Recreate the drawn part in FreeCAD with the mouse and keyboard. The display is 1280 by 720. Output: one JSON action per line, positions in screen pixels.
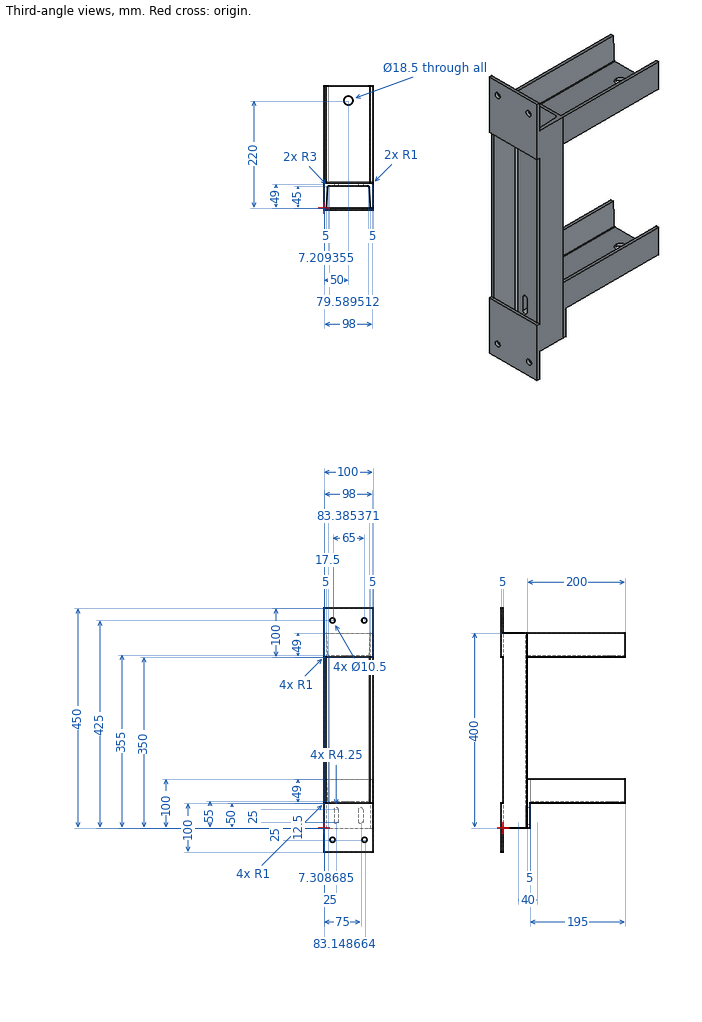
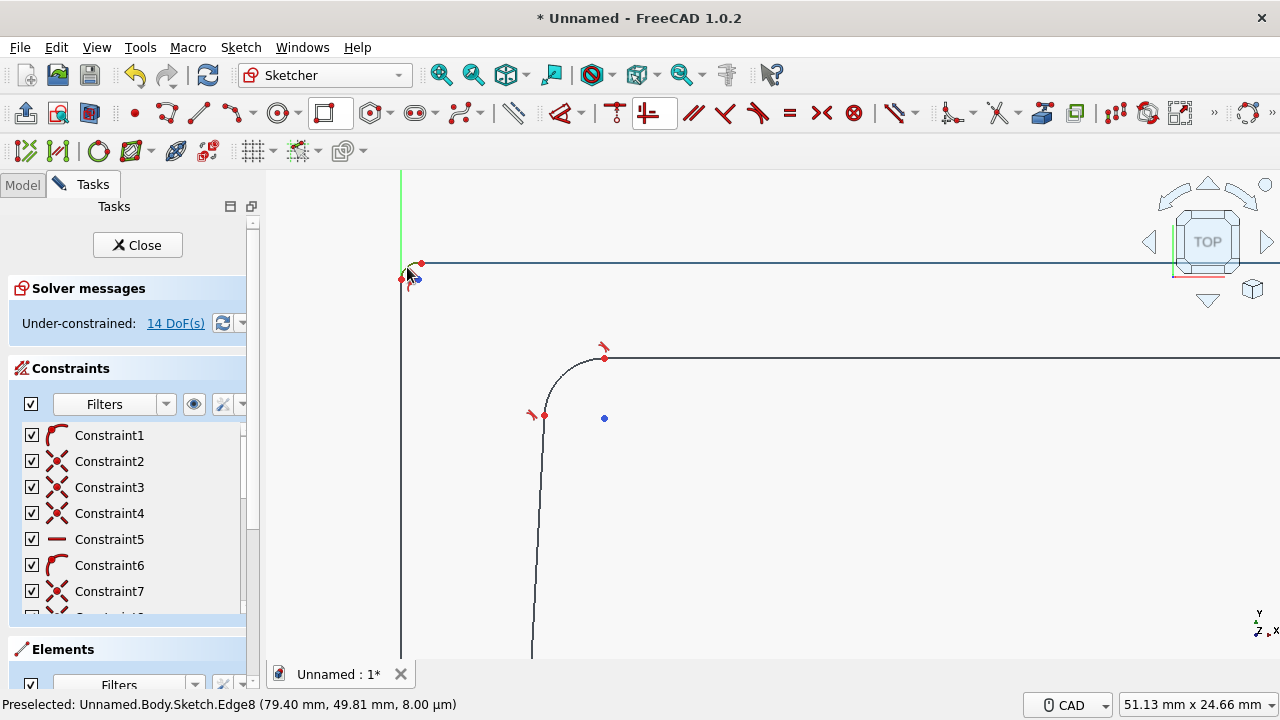
{"action": "left_click", "coordinate": [758, 114]}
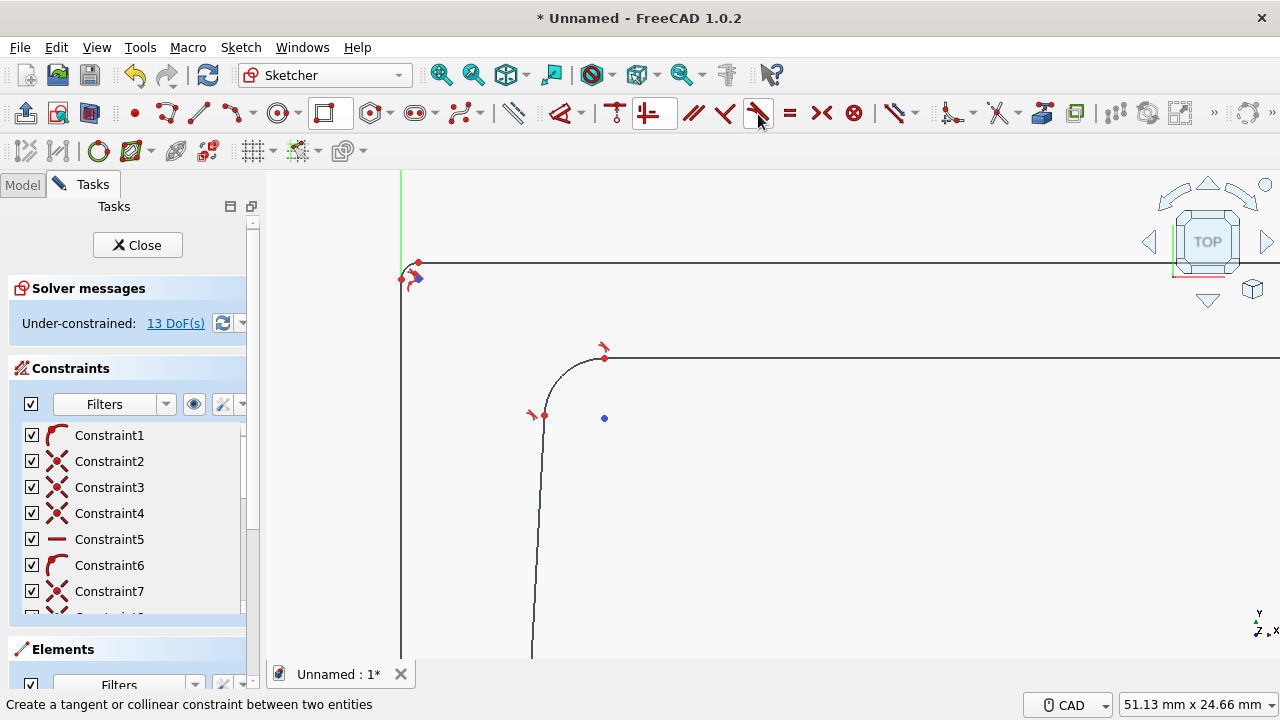
{"action": "scroll", "coordinate": [408, 268], "scroll_direction": "down", "scroll_amount": 6}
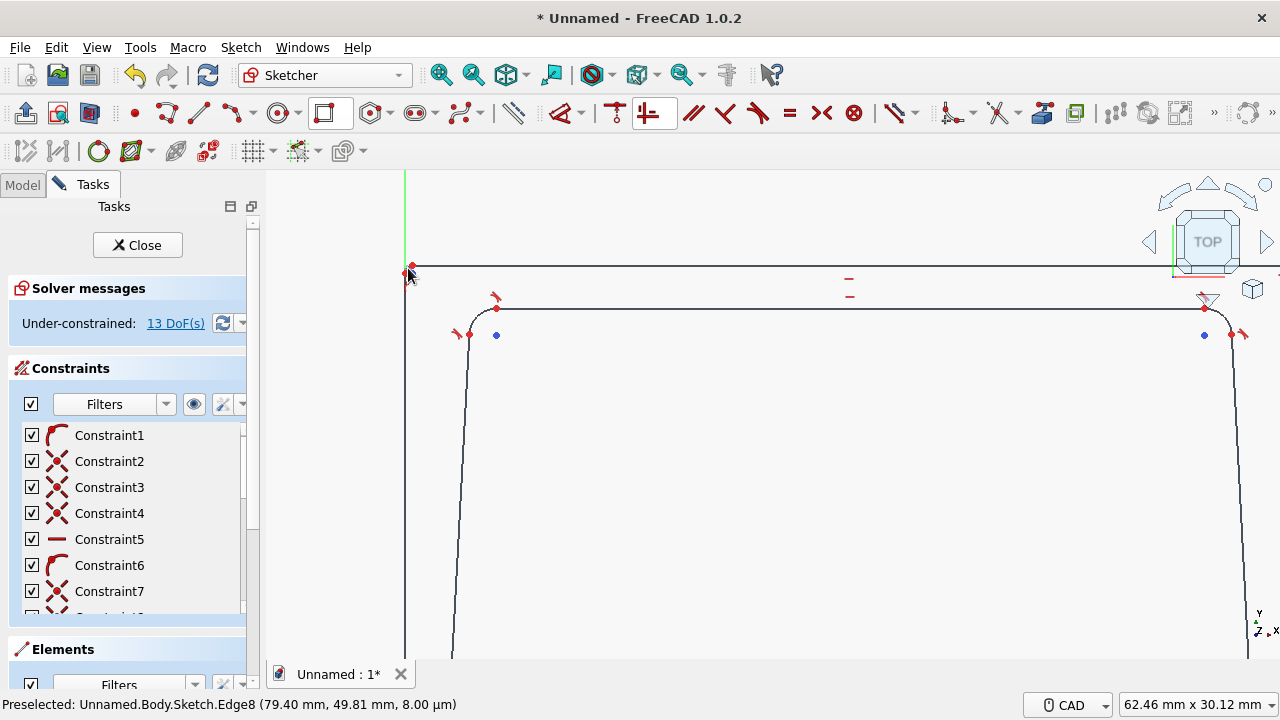
{"action": "scroll", "coordinate": [427, 559], "scroll_direction": "up", "scroll_amount": 5}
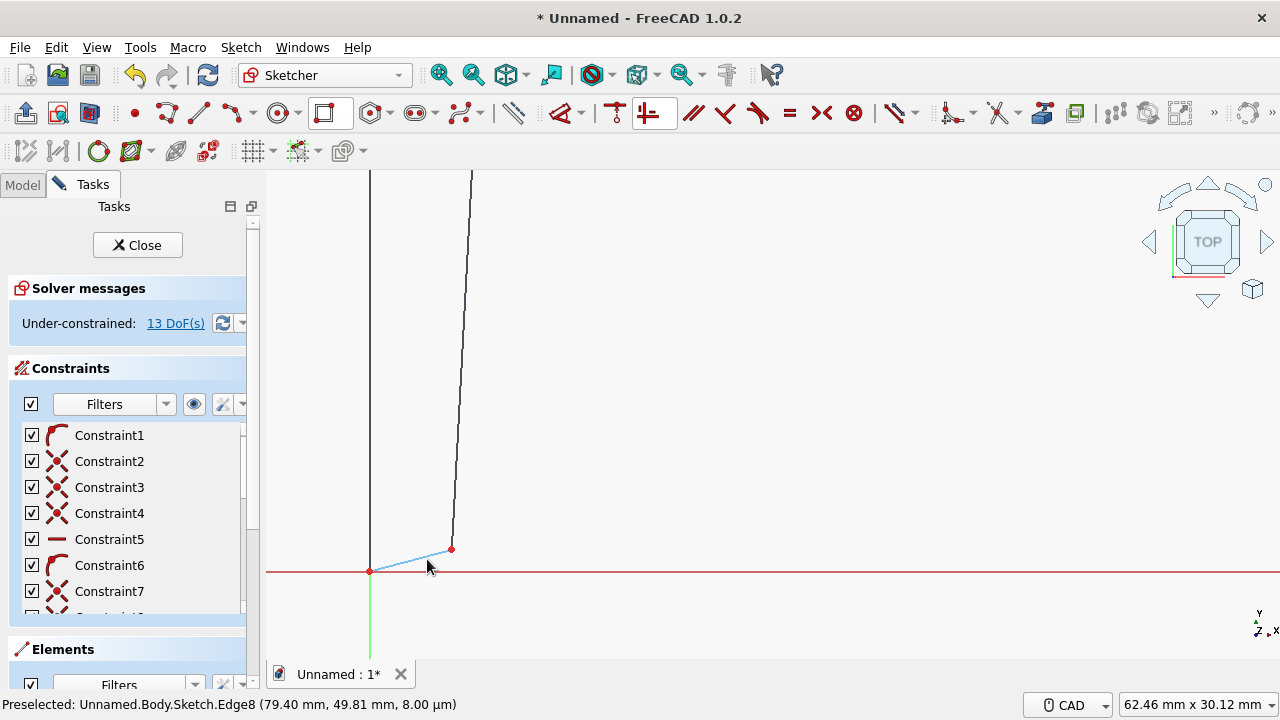
{"action": "left_click", "coordinate": [427, 556]}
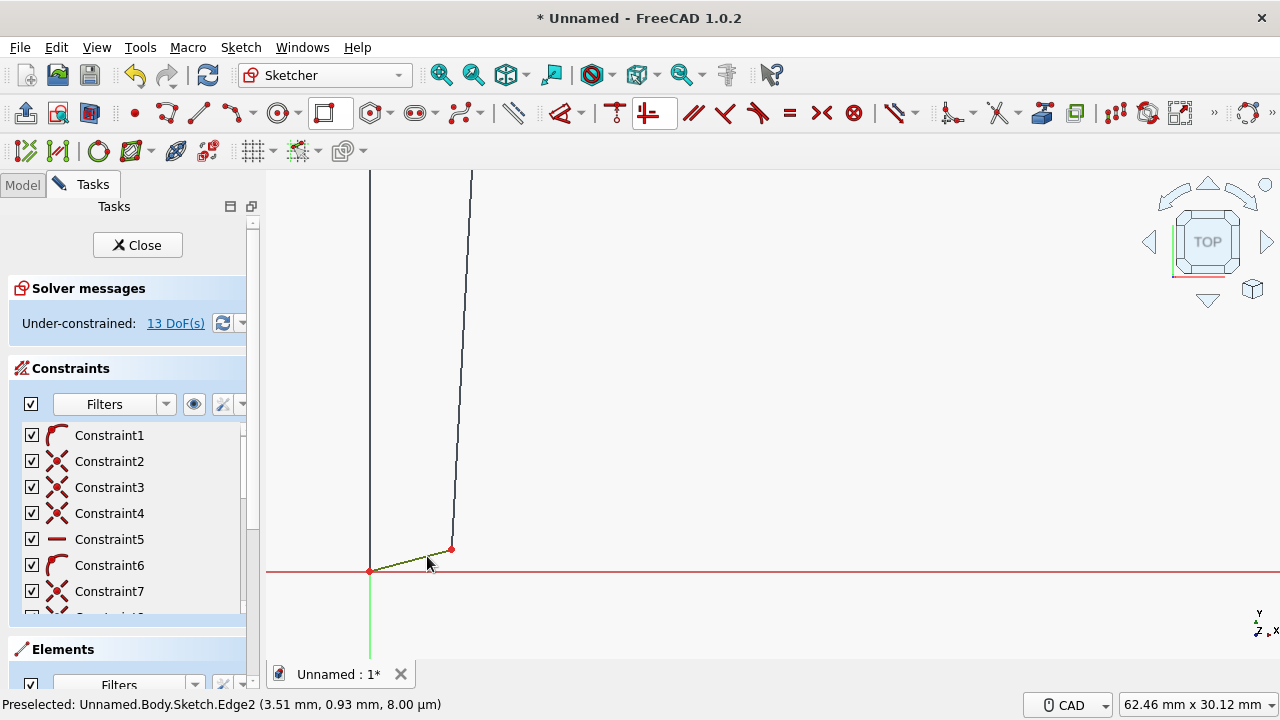
{"action": "left_click", "coordinate": [672, 114]}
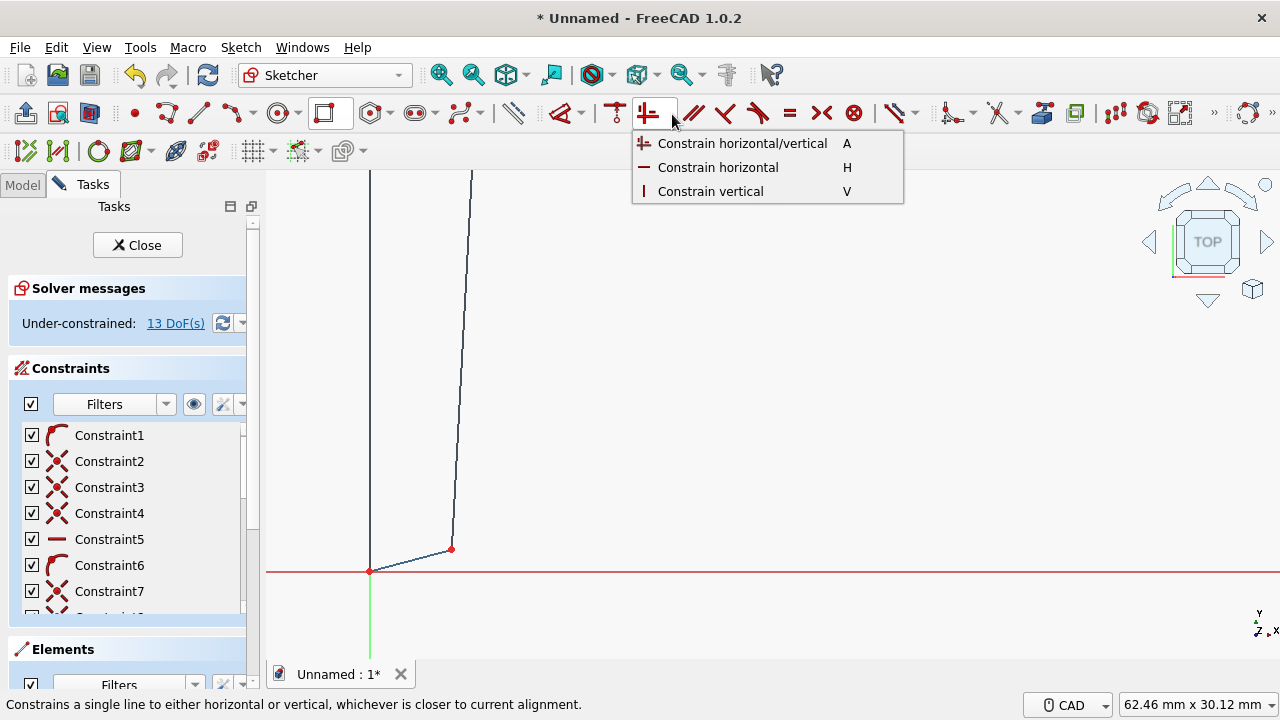
{"action": "left_click", "coordinate": [768, 167]}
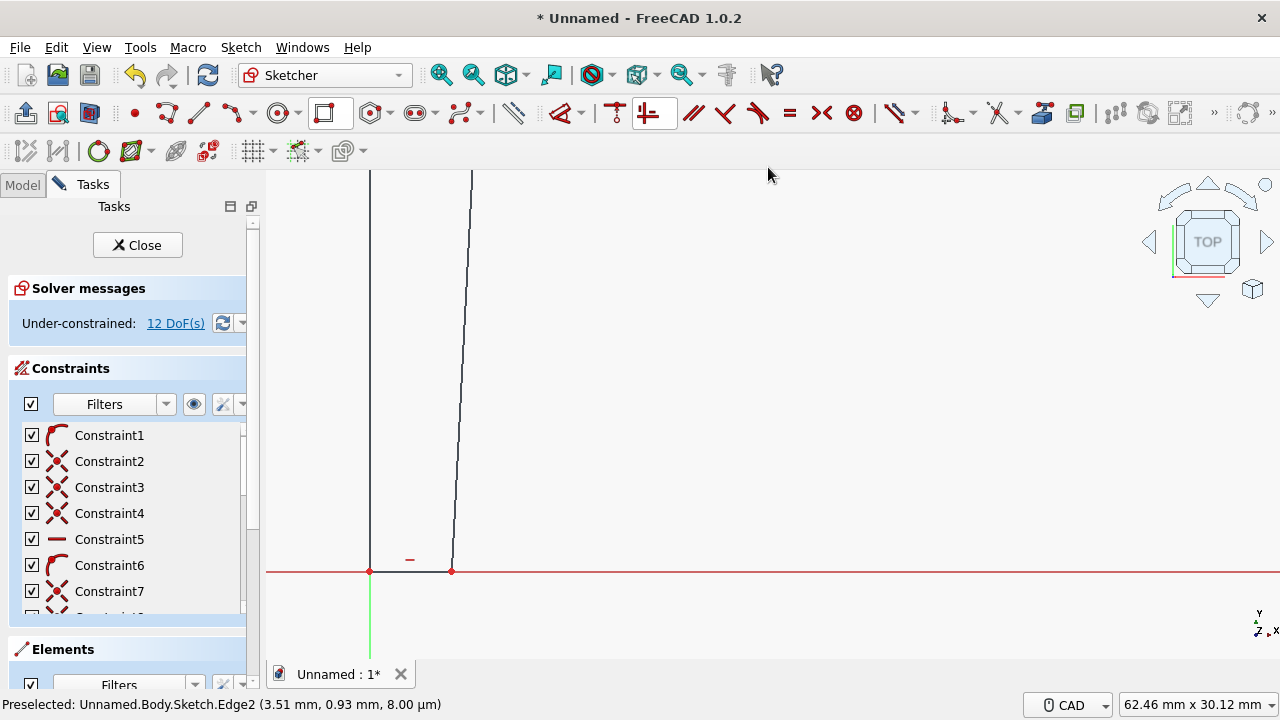
{"action": "scroll", "coordinate": [427, 559], "scroll_direction": "down", "scroll_amount": 5}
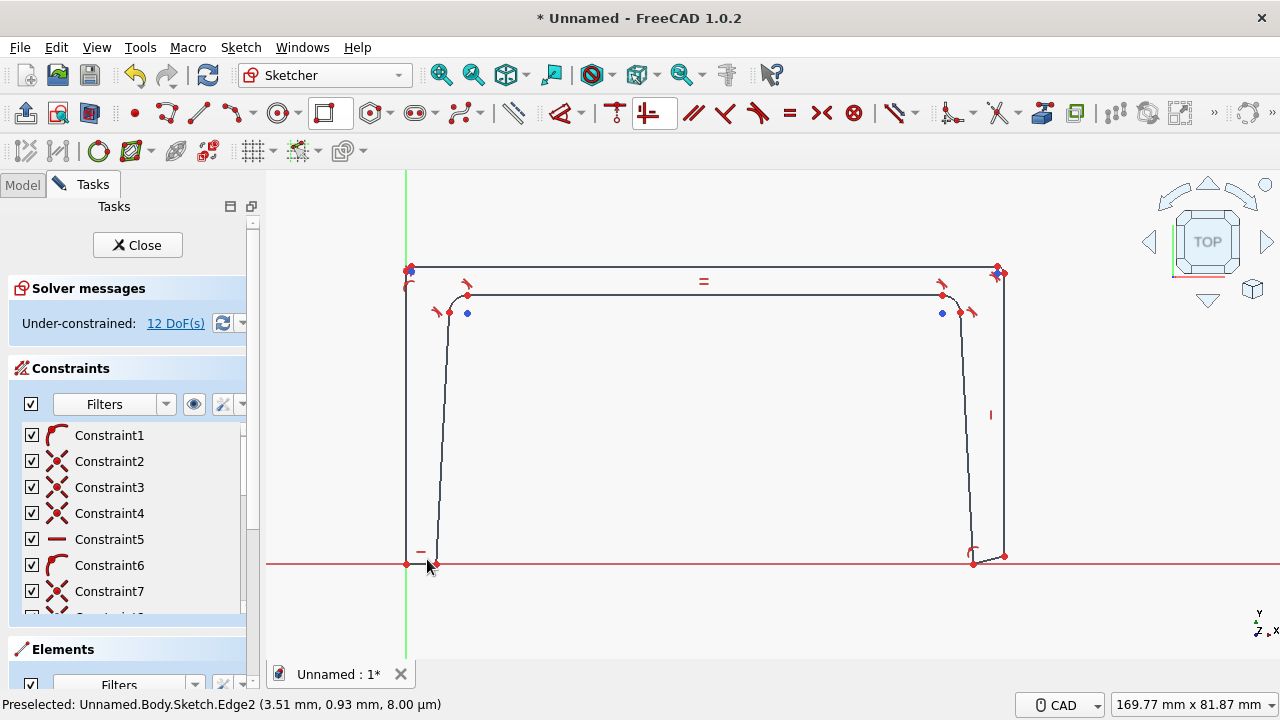
{"action": "scroll", "coordinate": [995, 559], "scroll_direction": "up", "scroll_amount": 5}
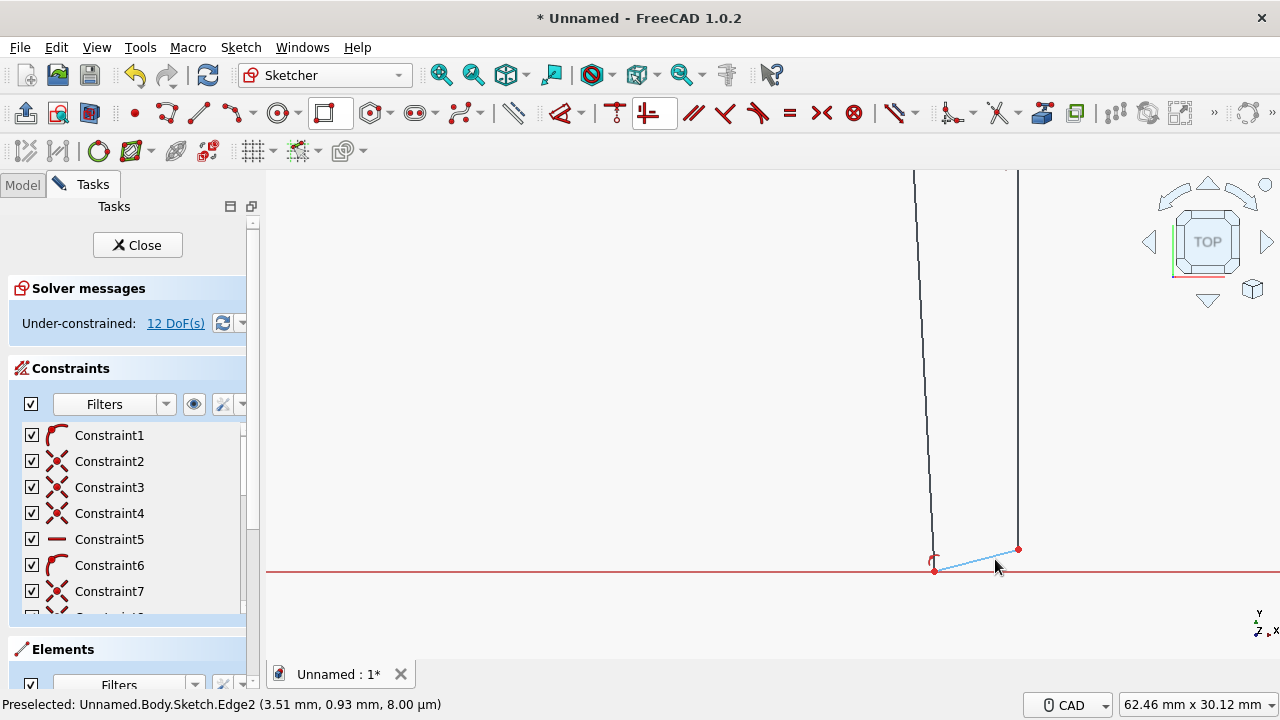
{"action": "left_click", "coordinate": [993, 556]}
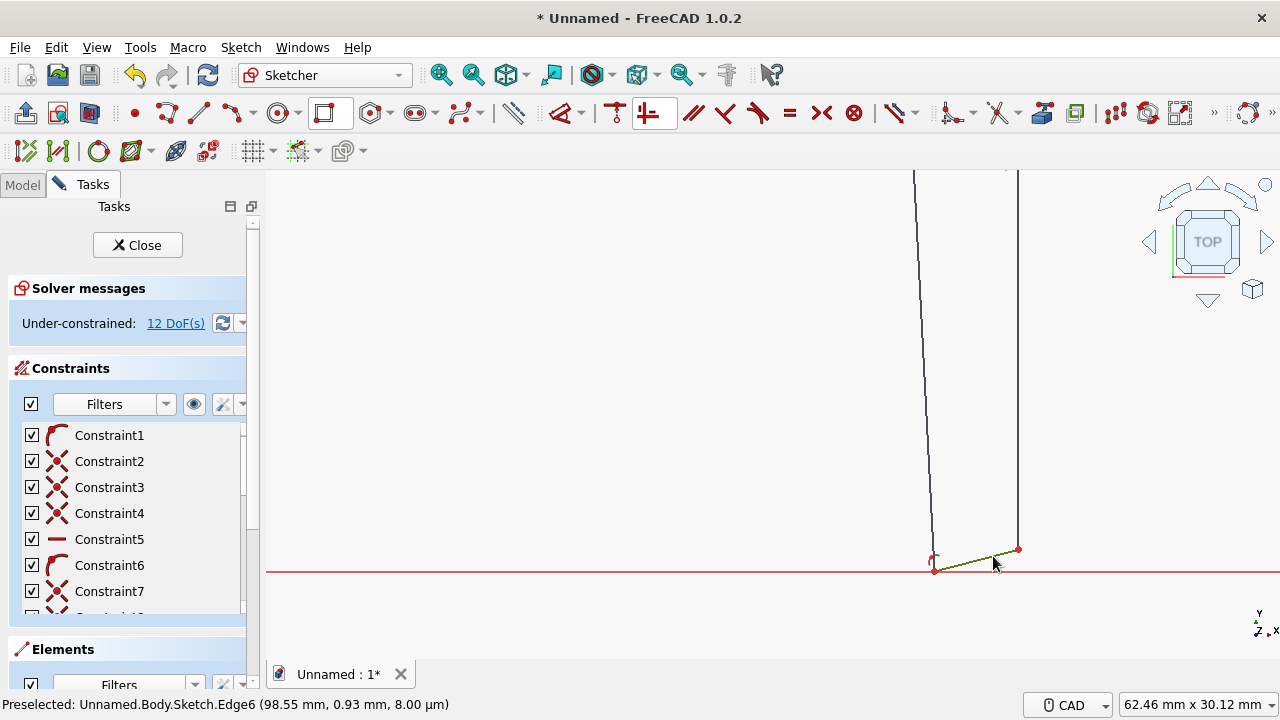
{"action": "left_click", "coordinate": [672, 114]}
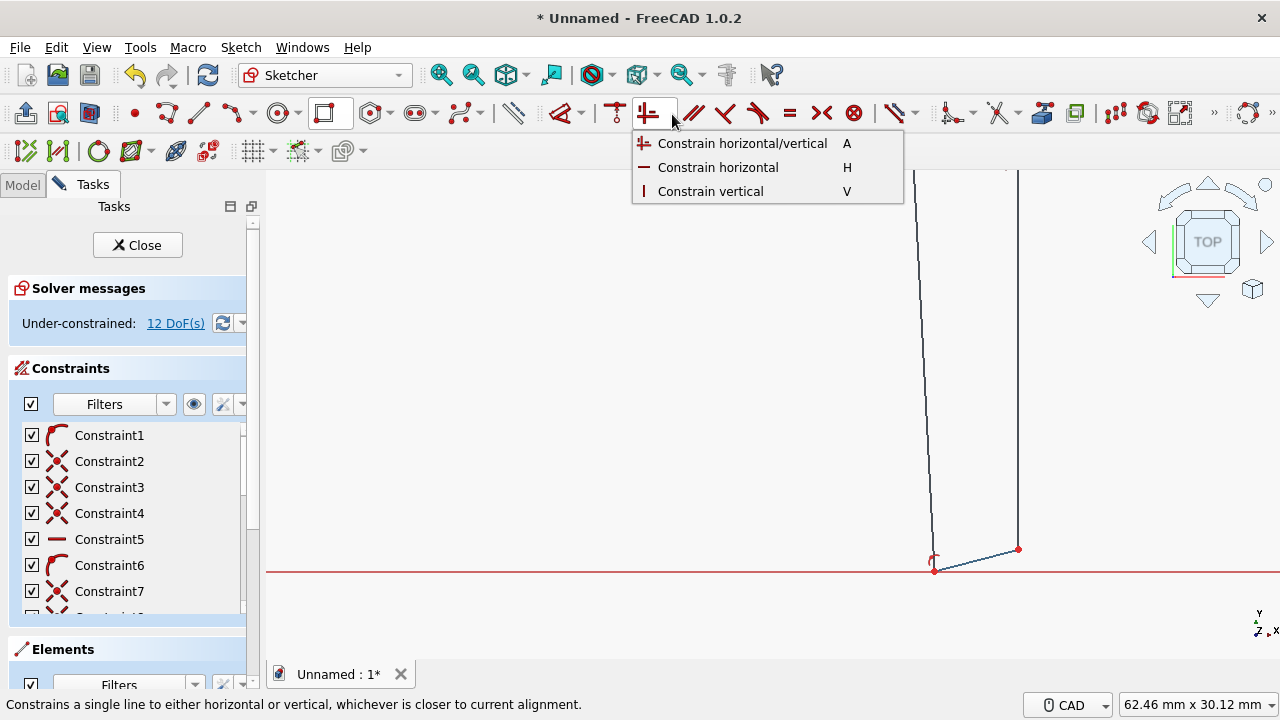
{"action": "left_click", "coordinate": [768, 167]}